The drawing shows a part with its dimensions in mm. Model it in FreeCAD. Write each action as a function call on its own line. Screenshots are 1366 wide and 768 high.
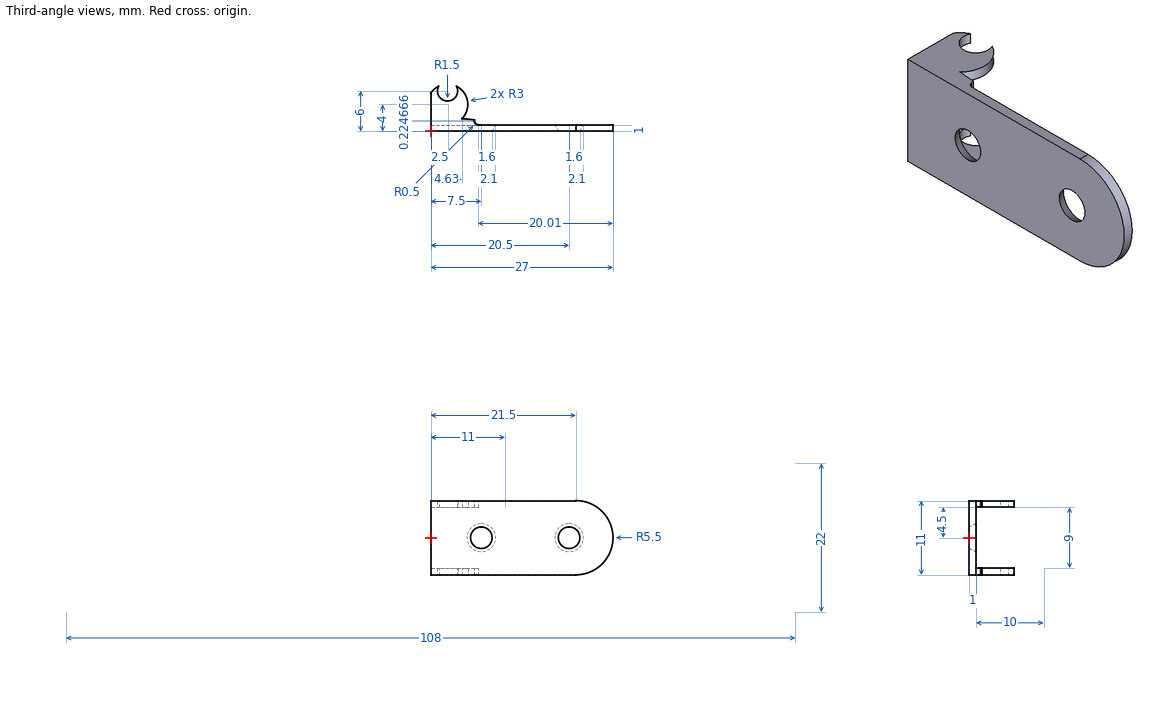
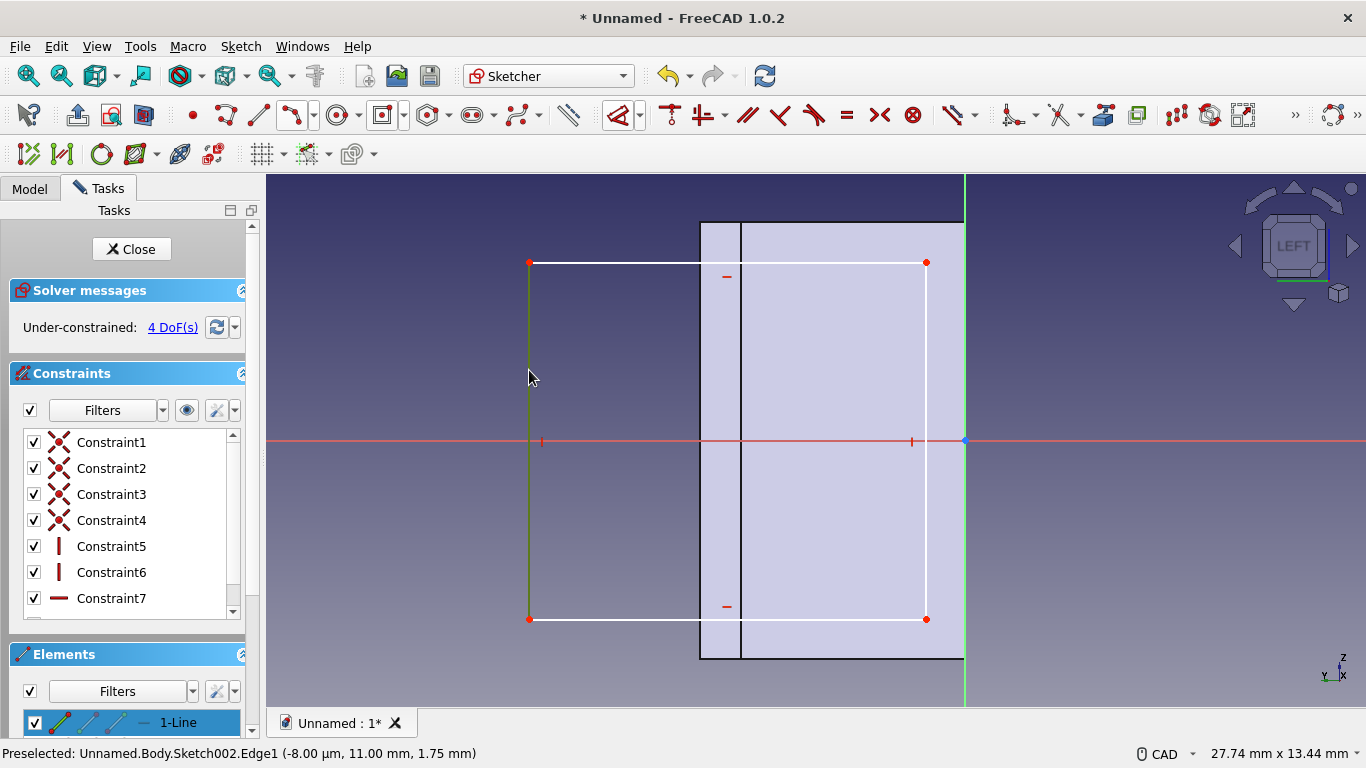
key(i)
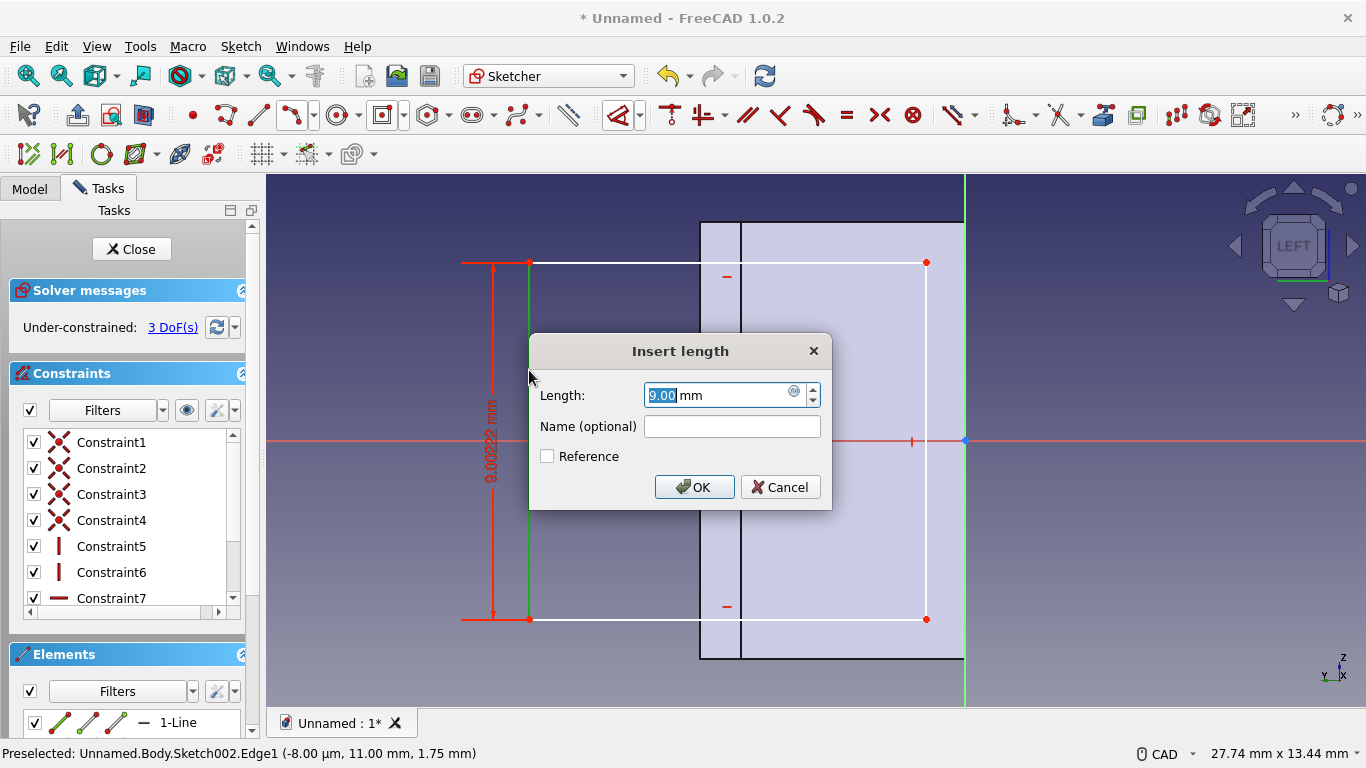
text(9)
key(Return)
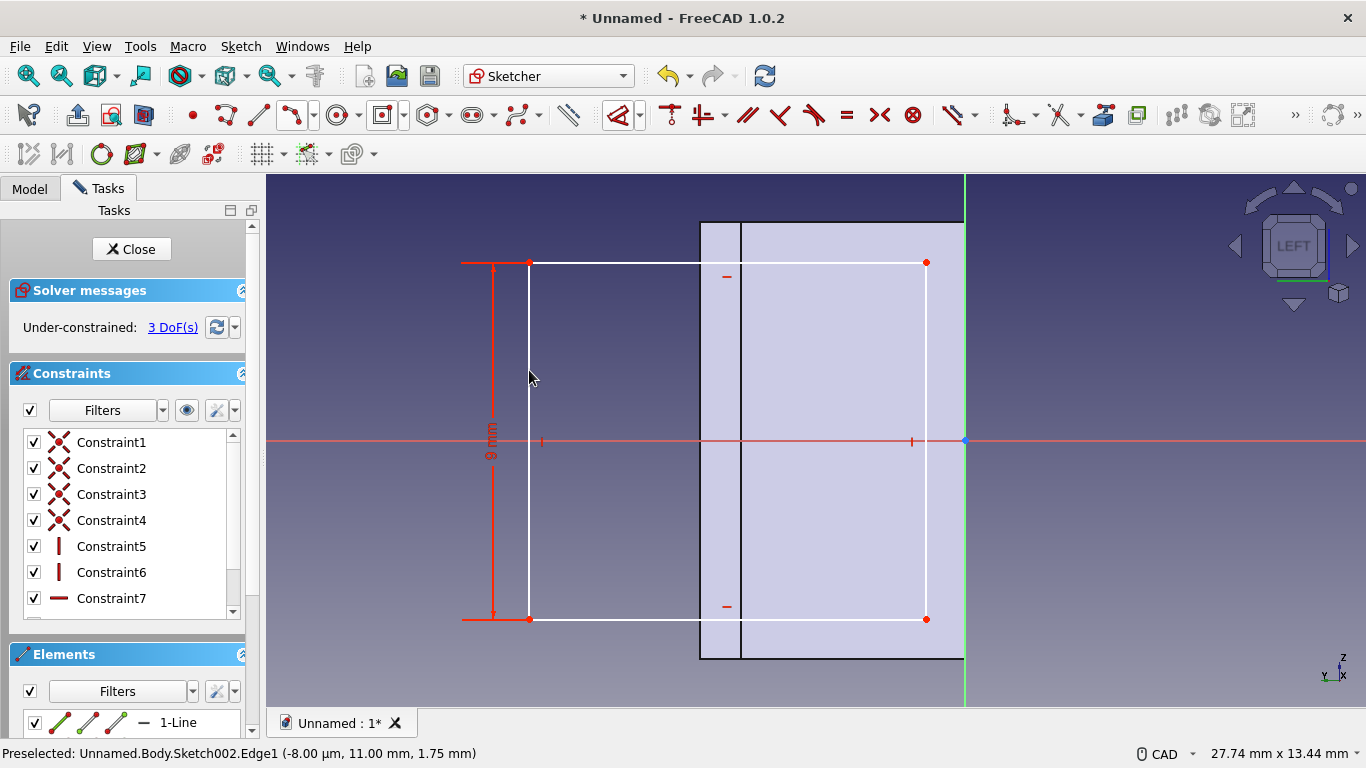
click(648, 620)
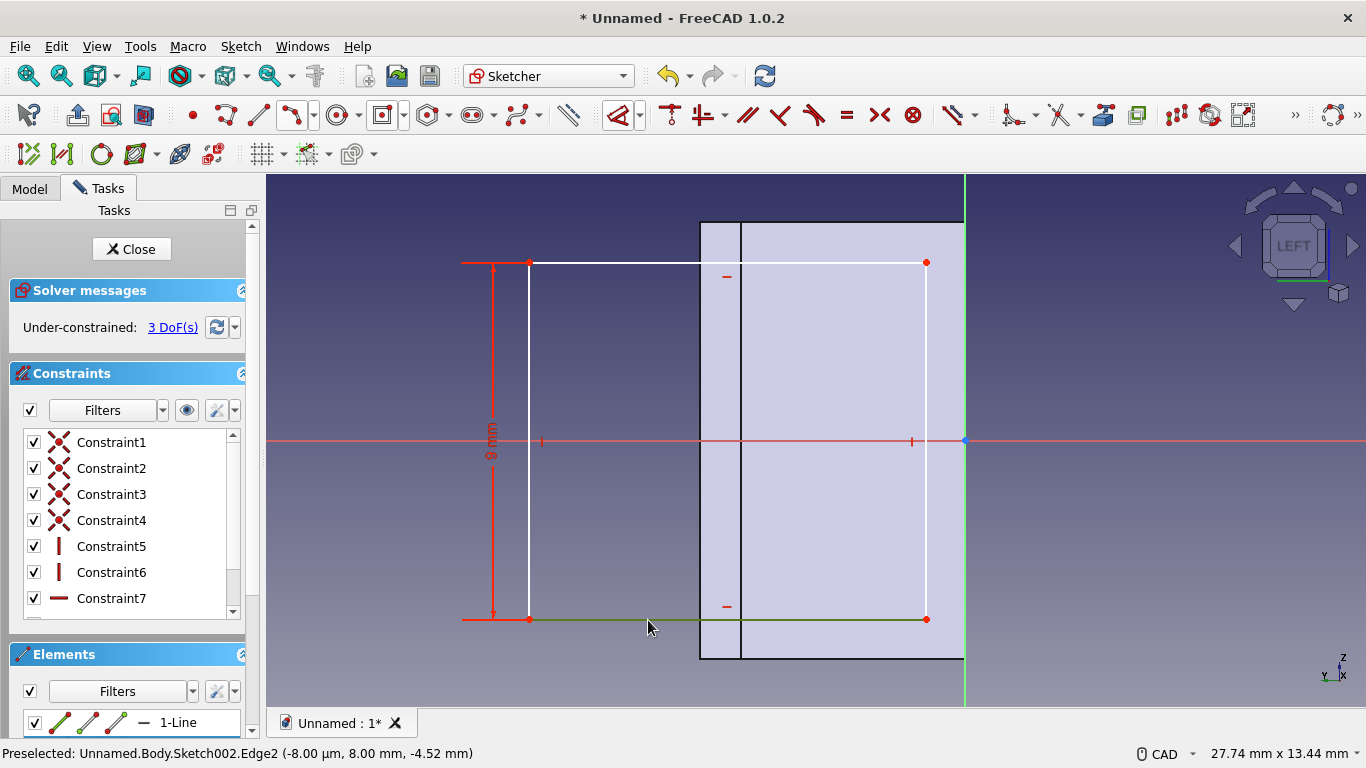
key(l)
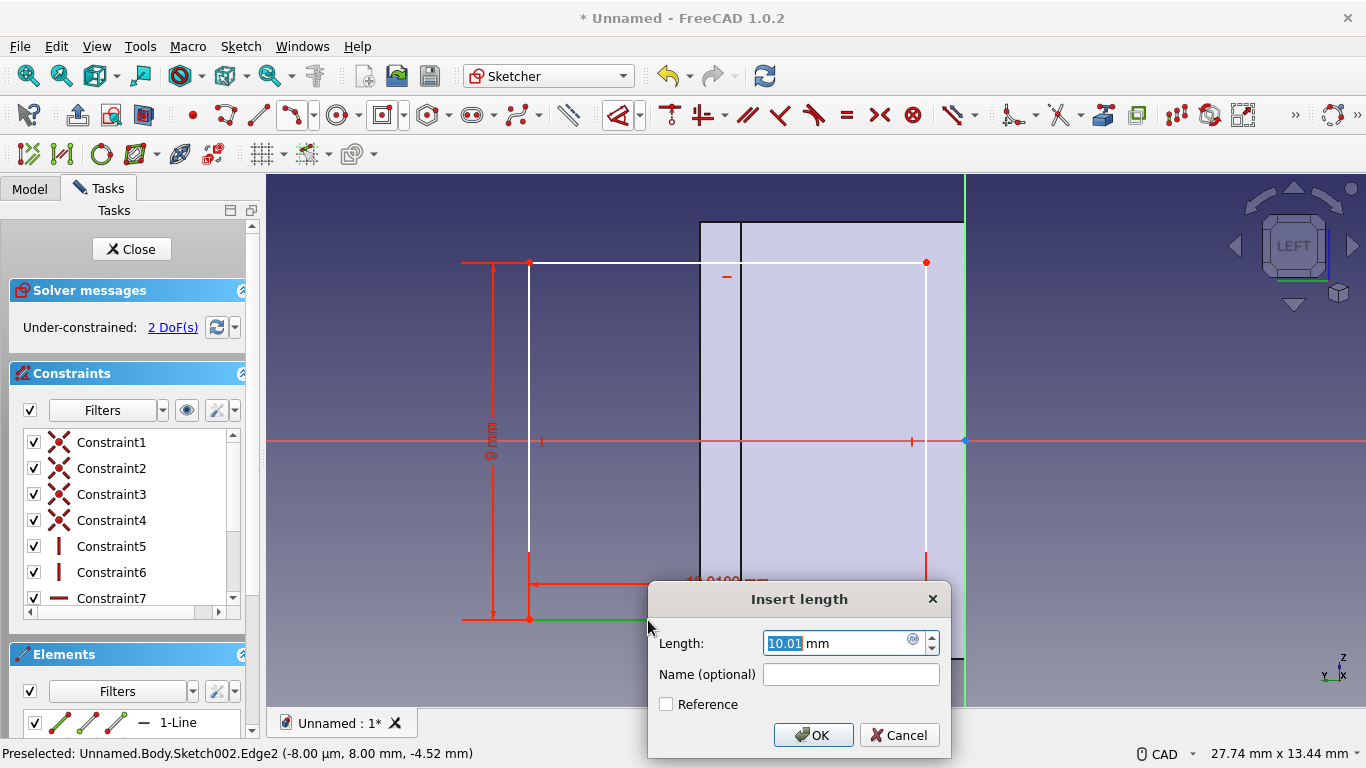
text(10)
key(Return)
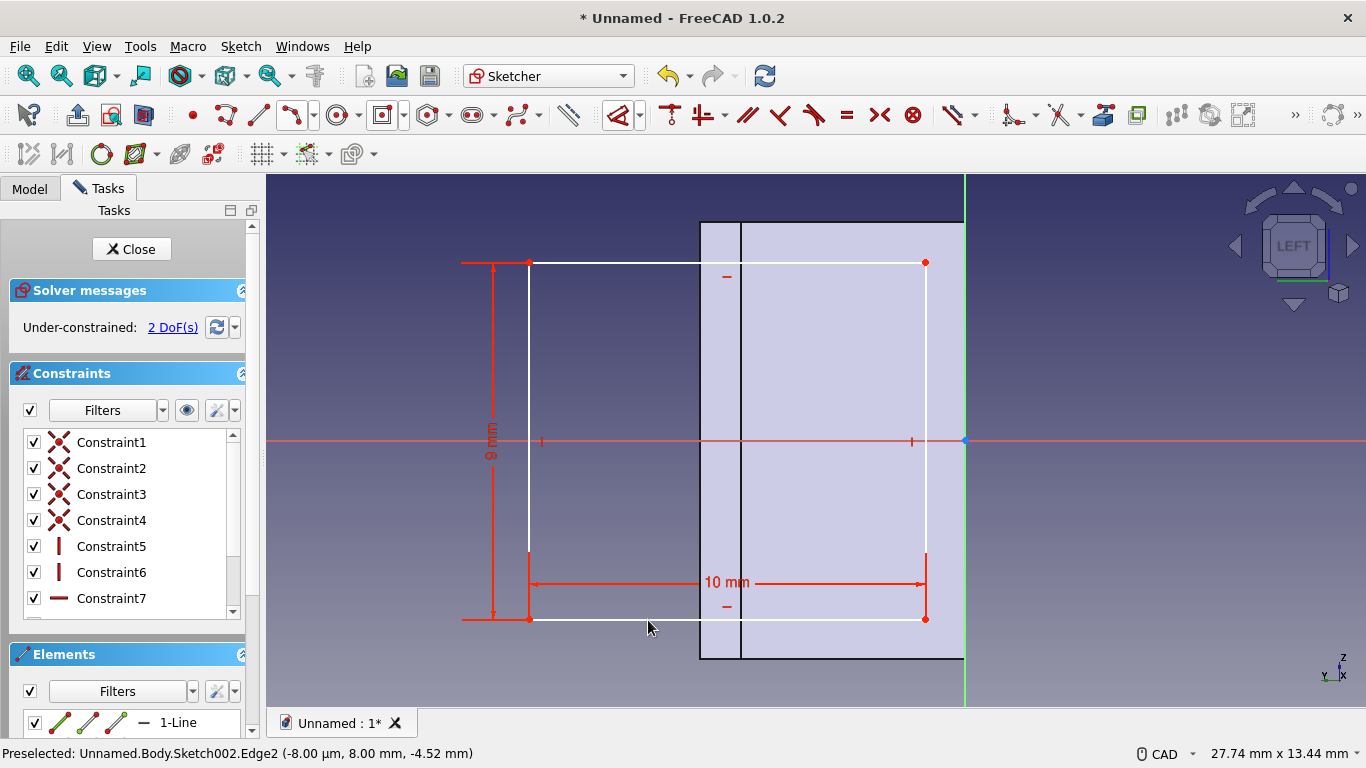
click(926, 620)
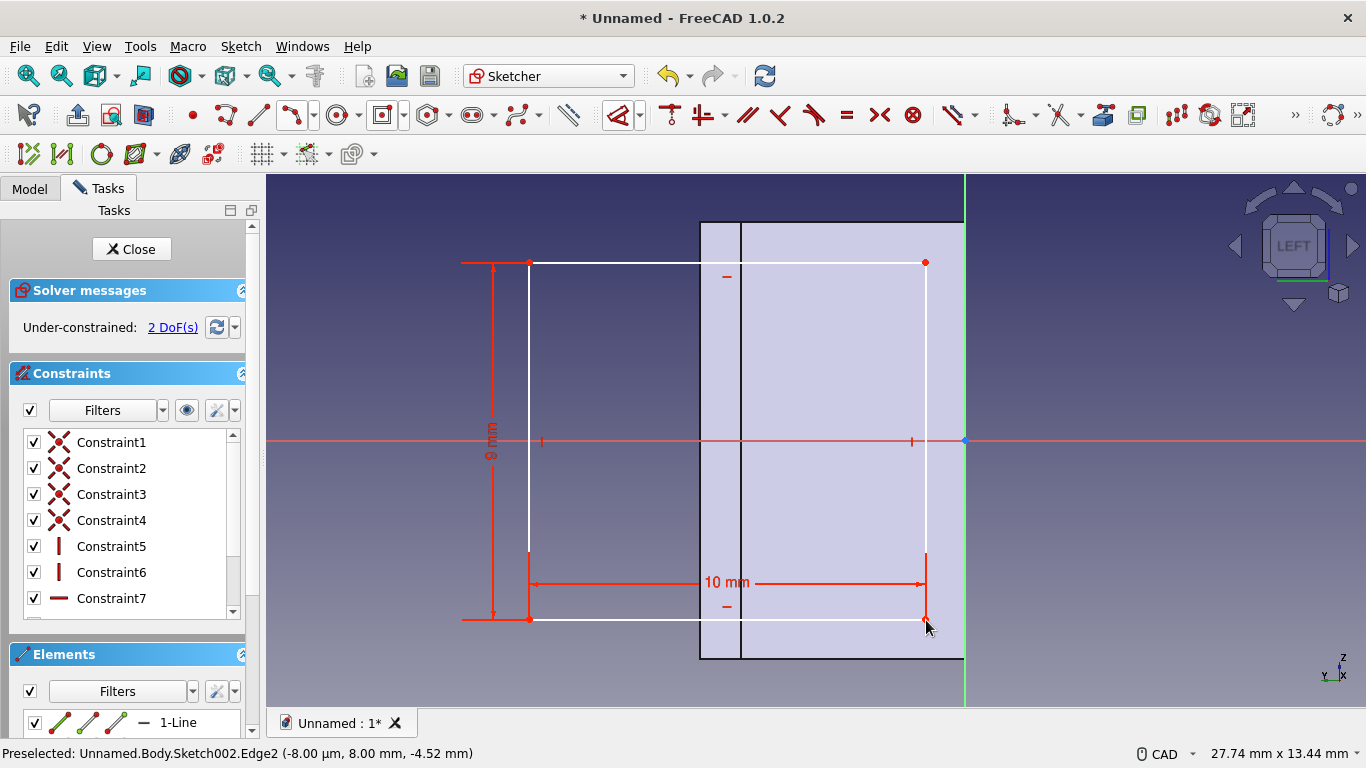
click(640, 116)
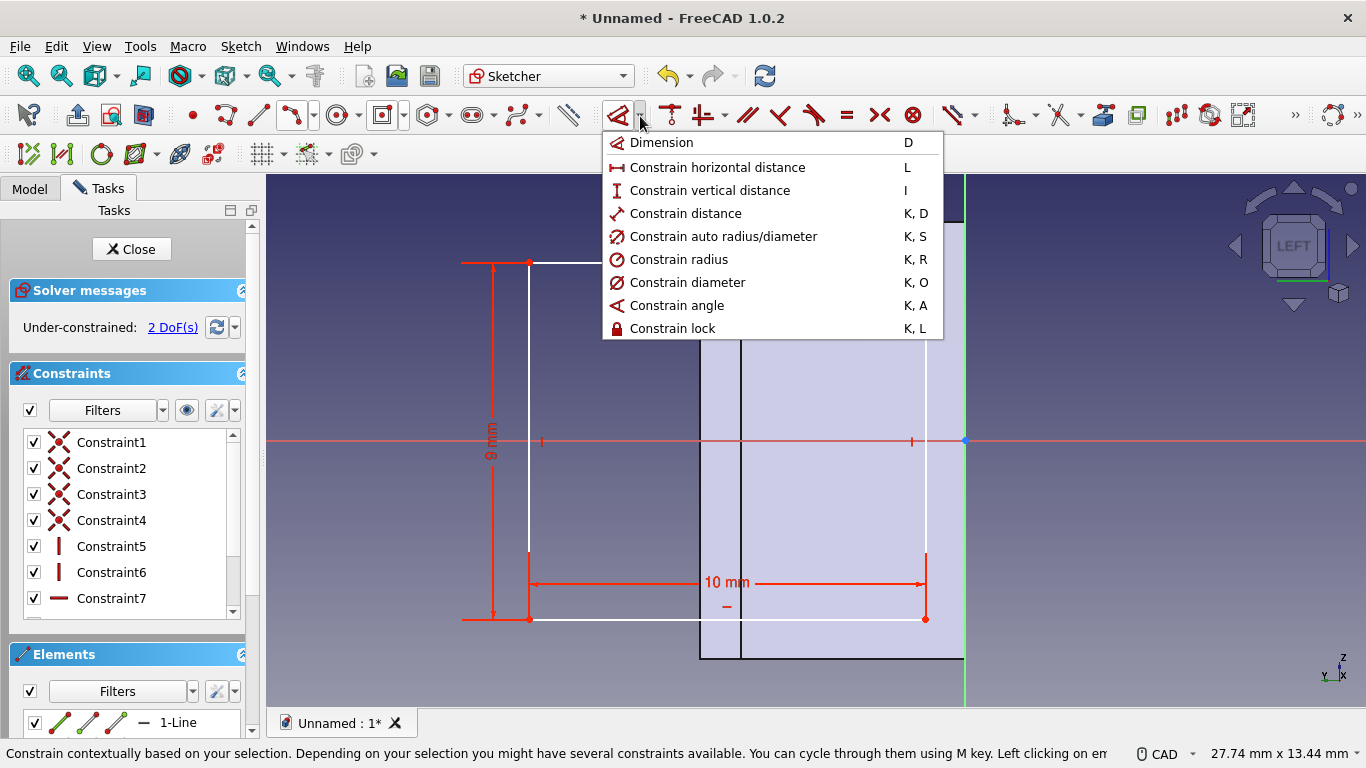
click(773, 168)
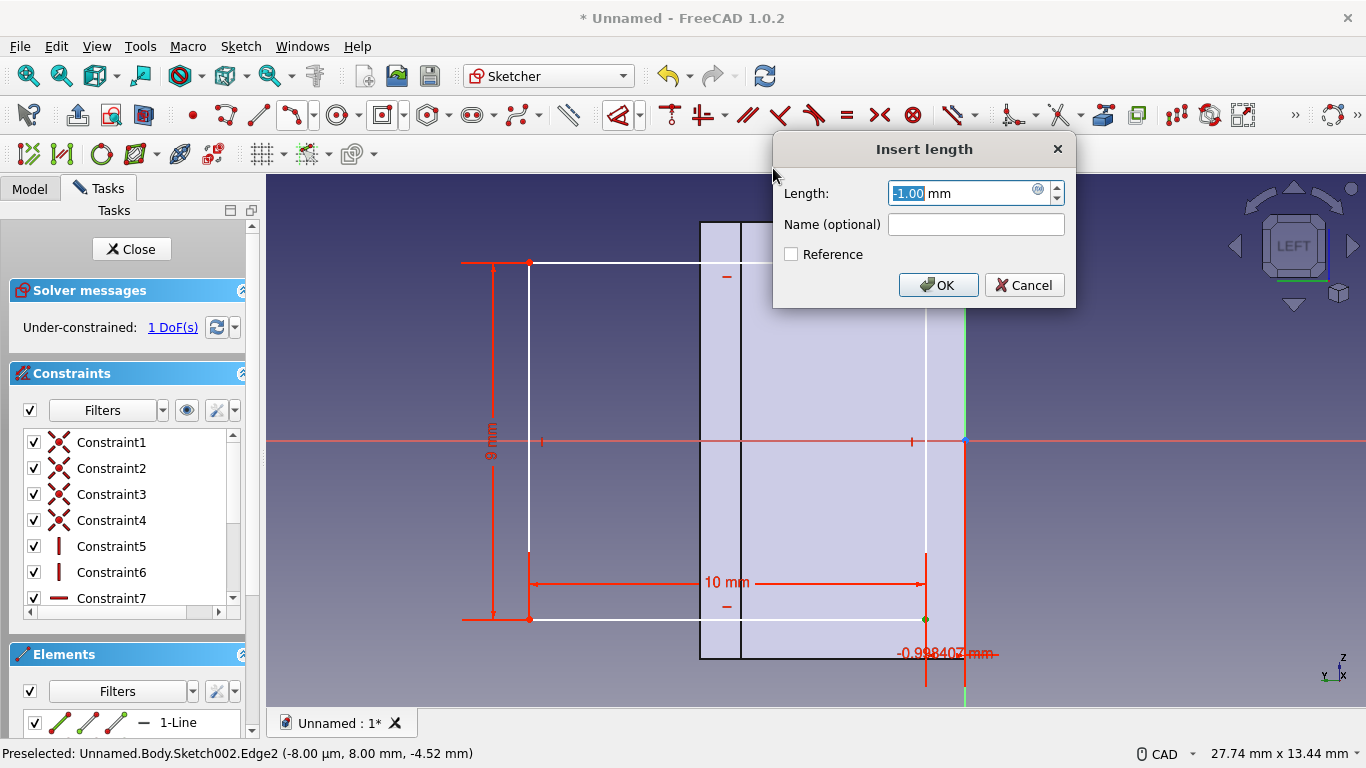
text(-1)
key(Return)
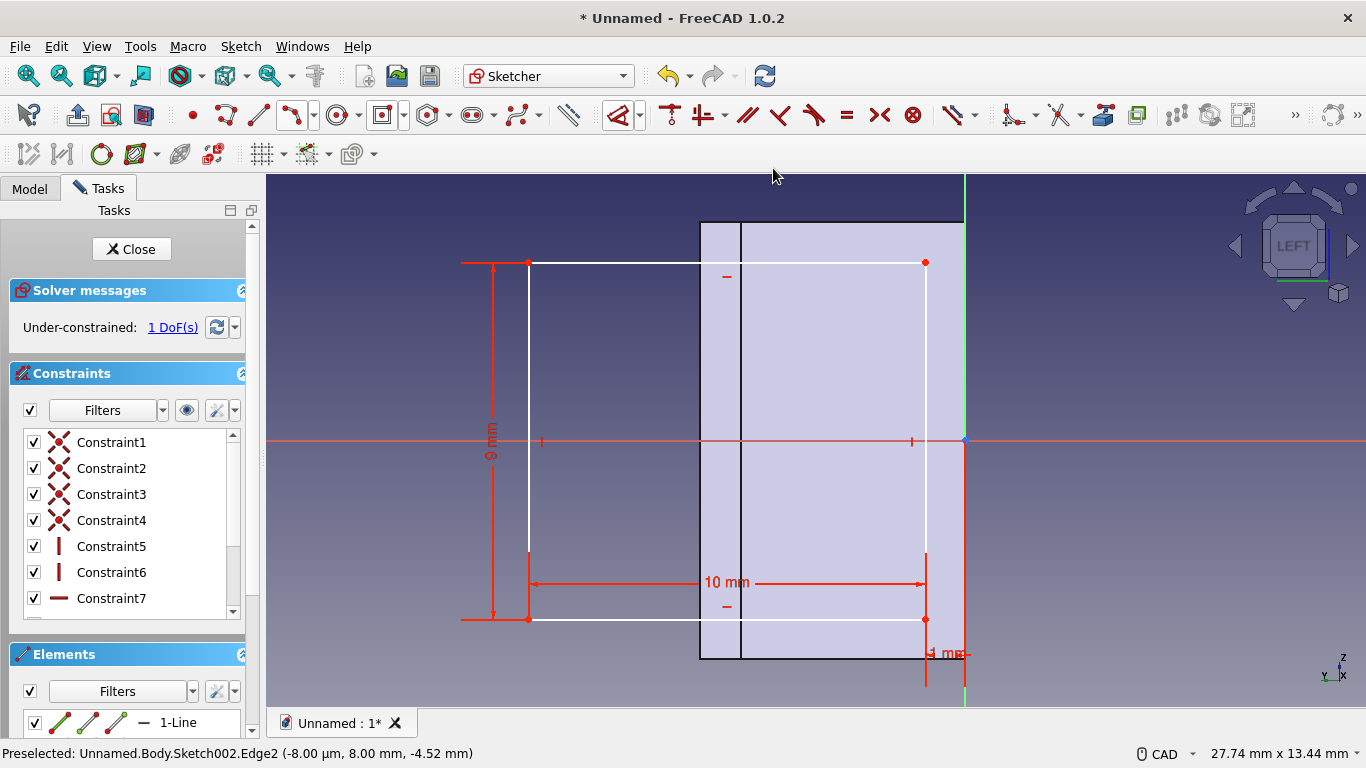
click(529, 263)